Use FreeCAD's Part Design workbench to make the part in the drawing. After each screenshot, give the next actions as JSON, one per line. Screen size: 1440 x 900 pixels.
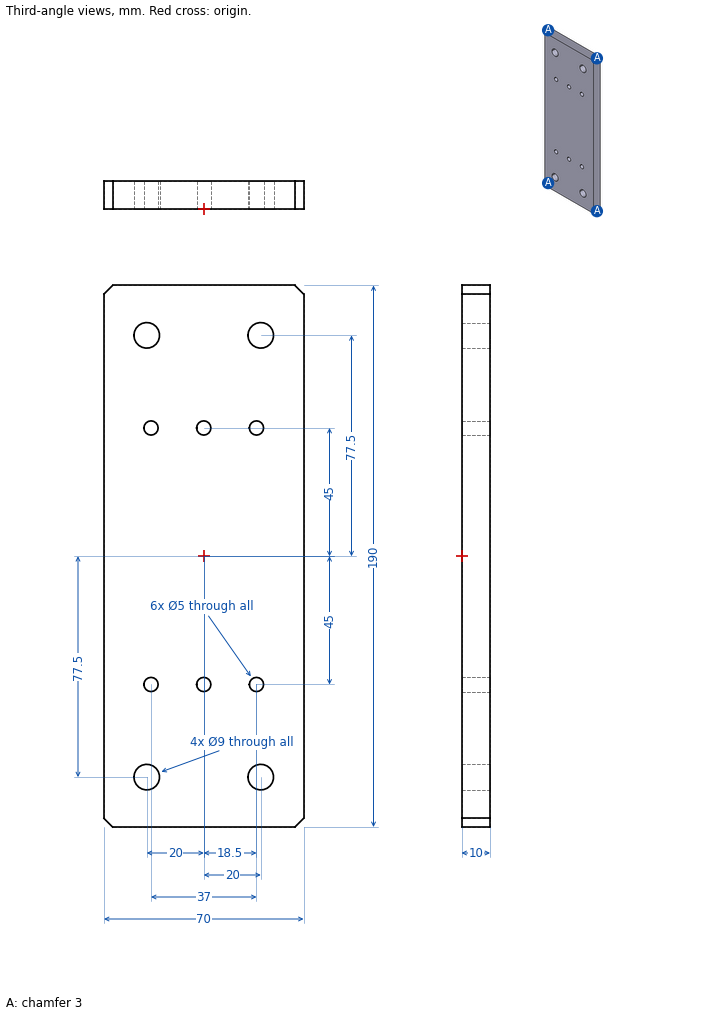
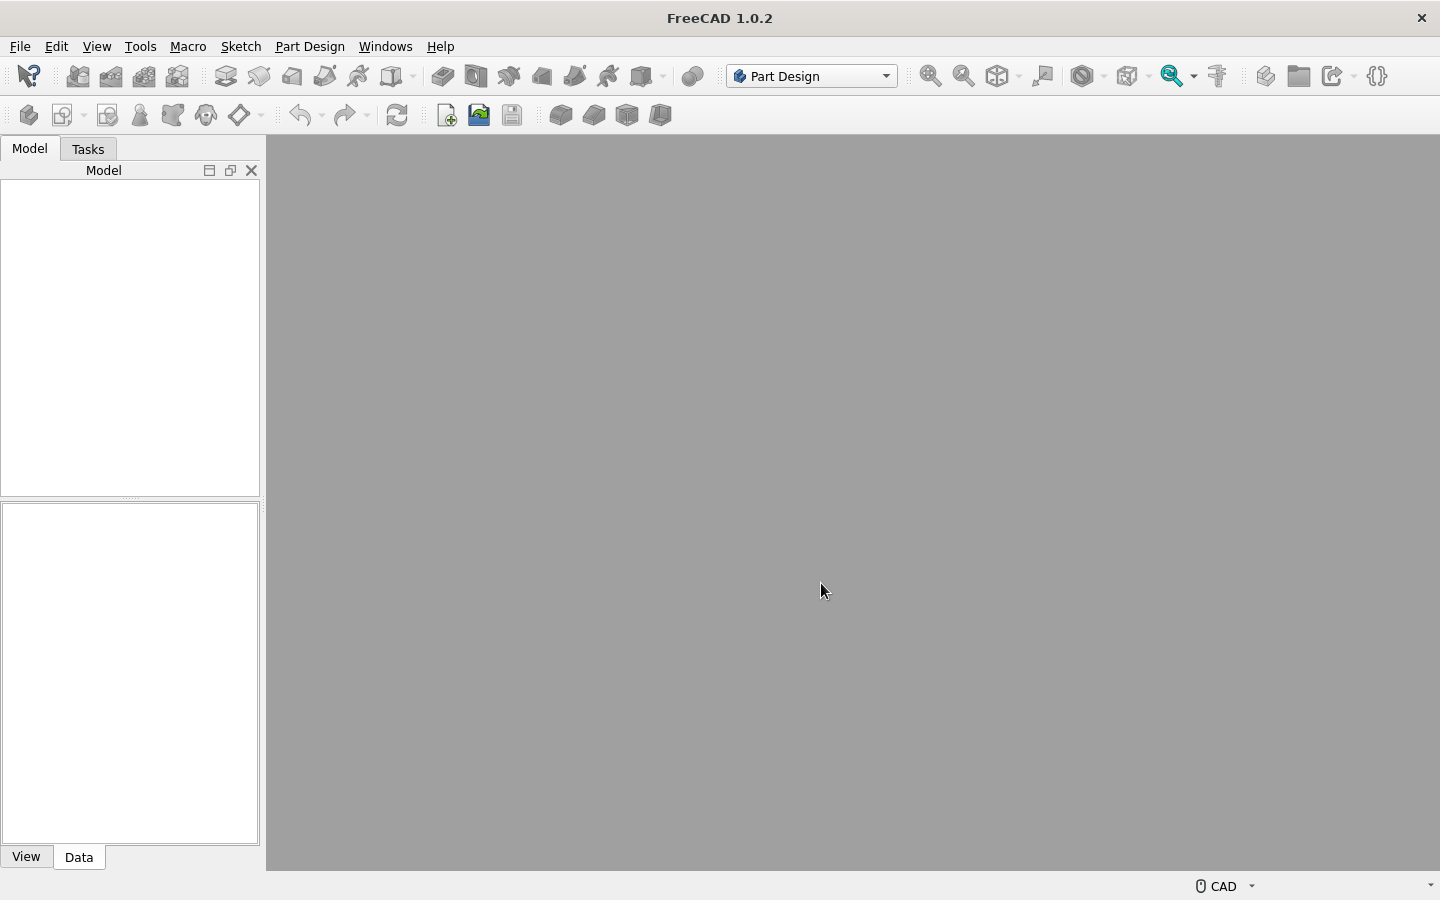
{"action": "left_click", "coordinate": [446, 116]}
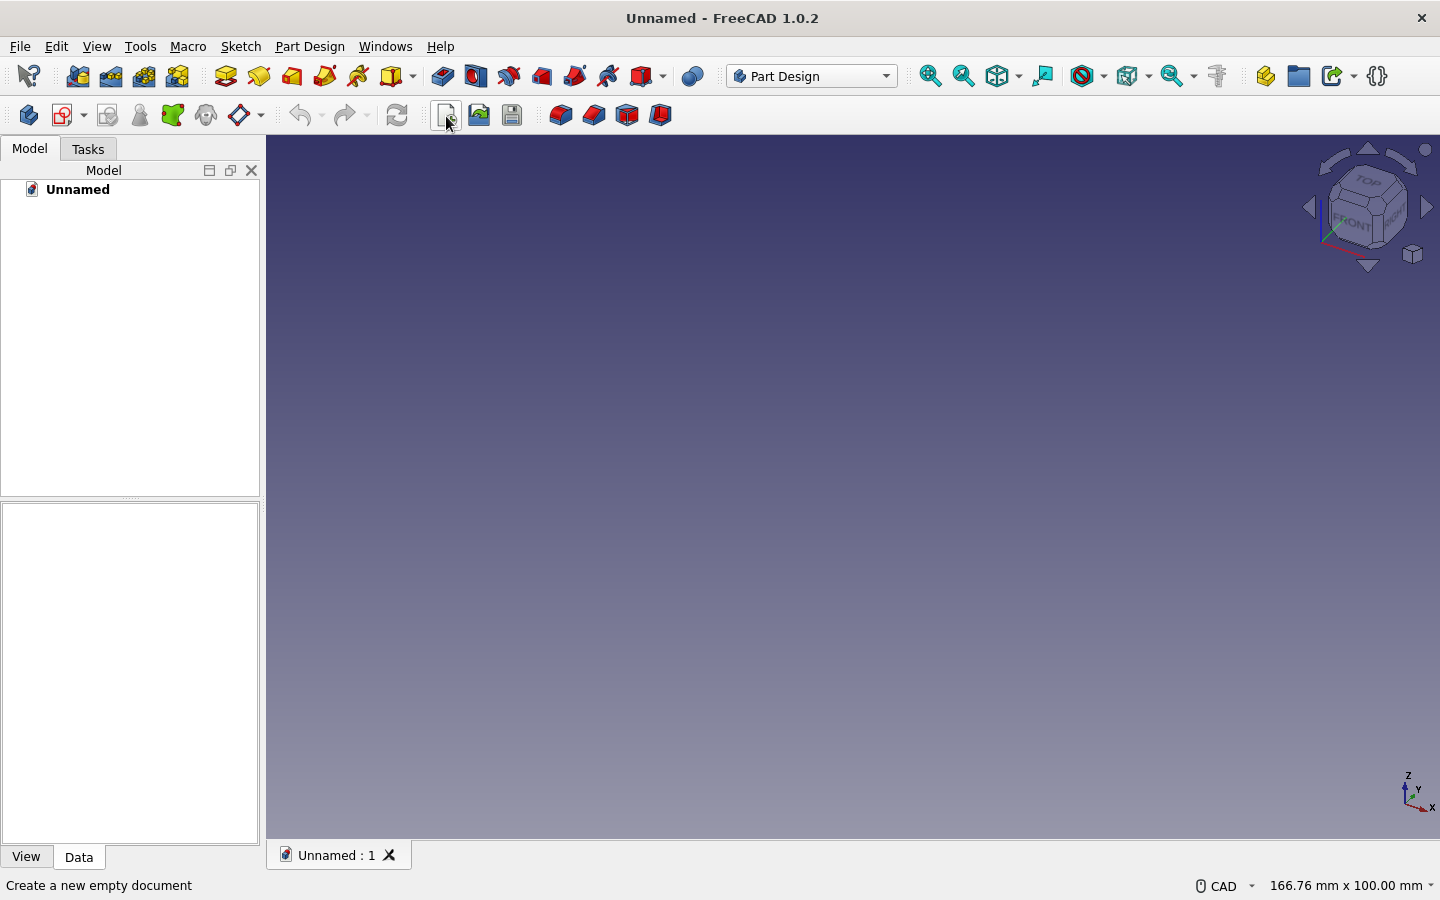
{"action": "left_click", "coordinate": [62, 116]}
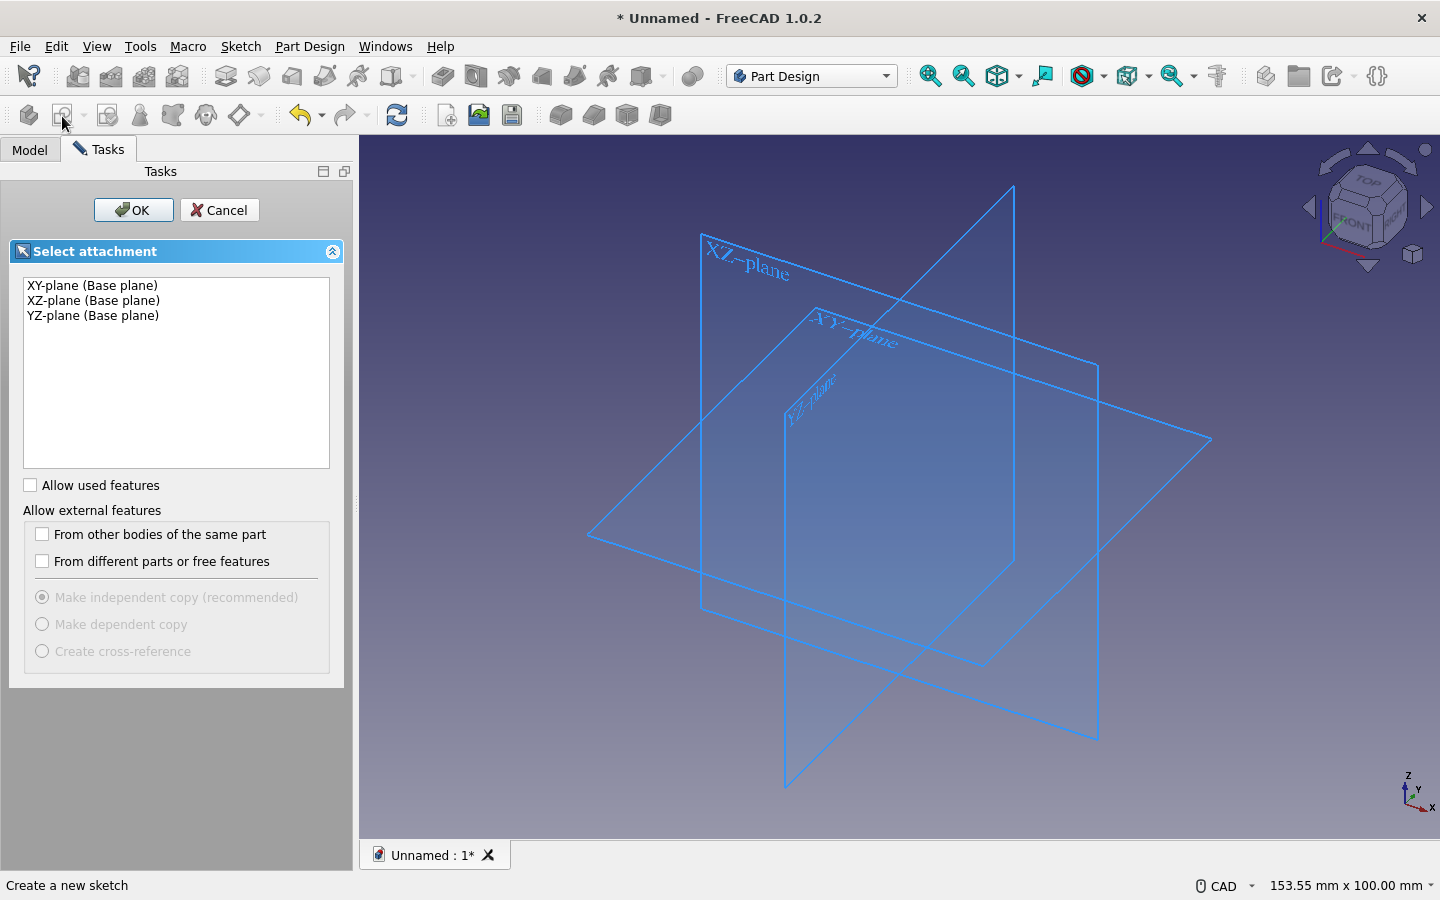
{"action": "left_click", "coordinate": [84, 300]}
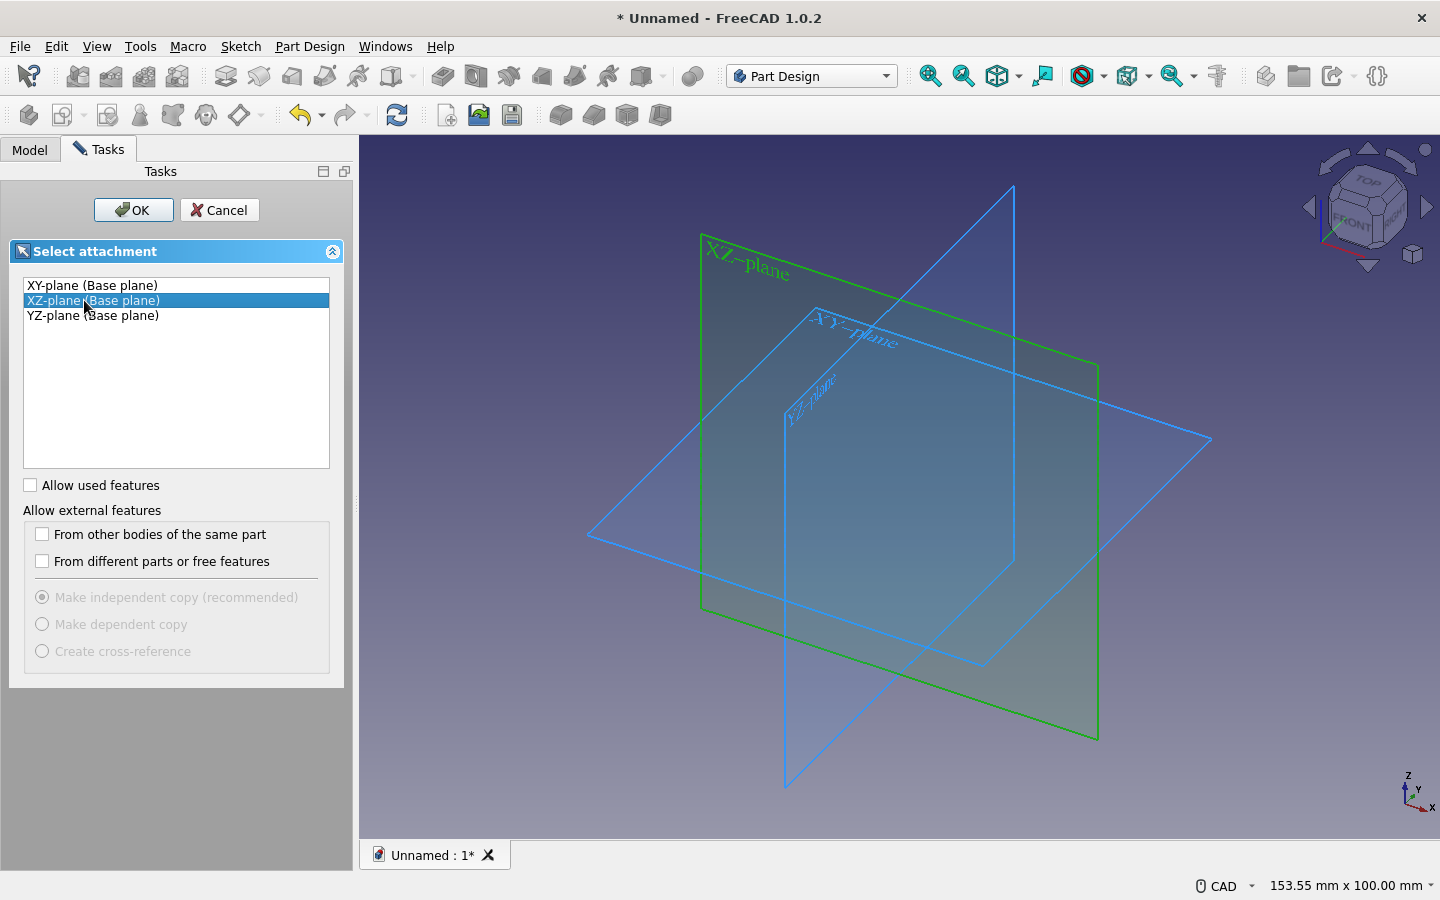
{"action": "left_click", "coordinate": [134, 210]}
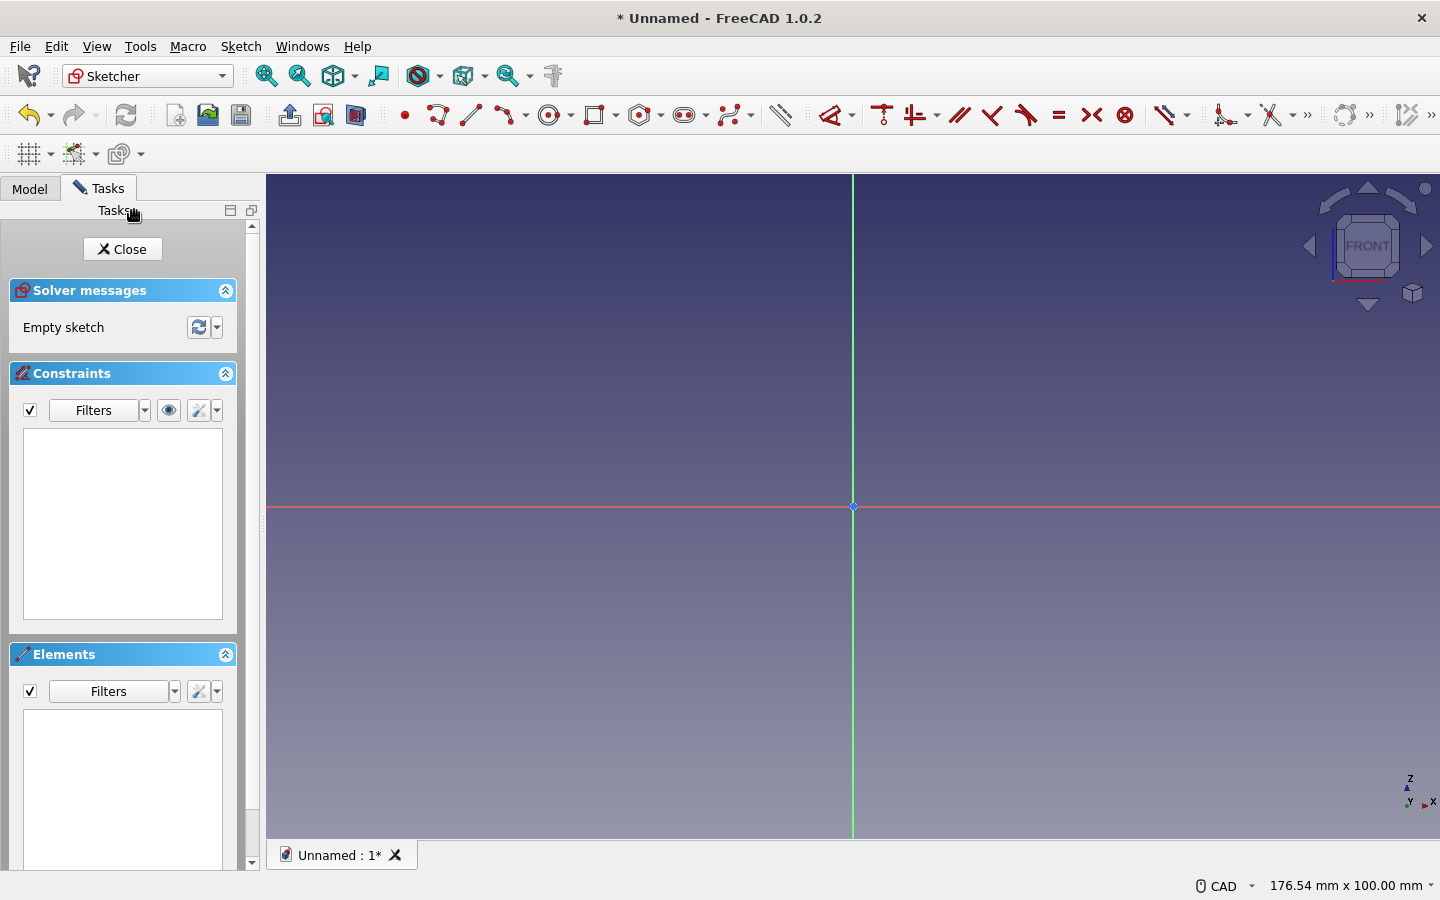
{"action": "scroll", "coordinate": [745, 506], "scroll_direction": "down", "scroll_amount": 5}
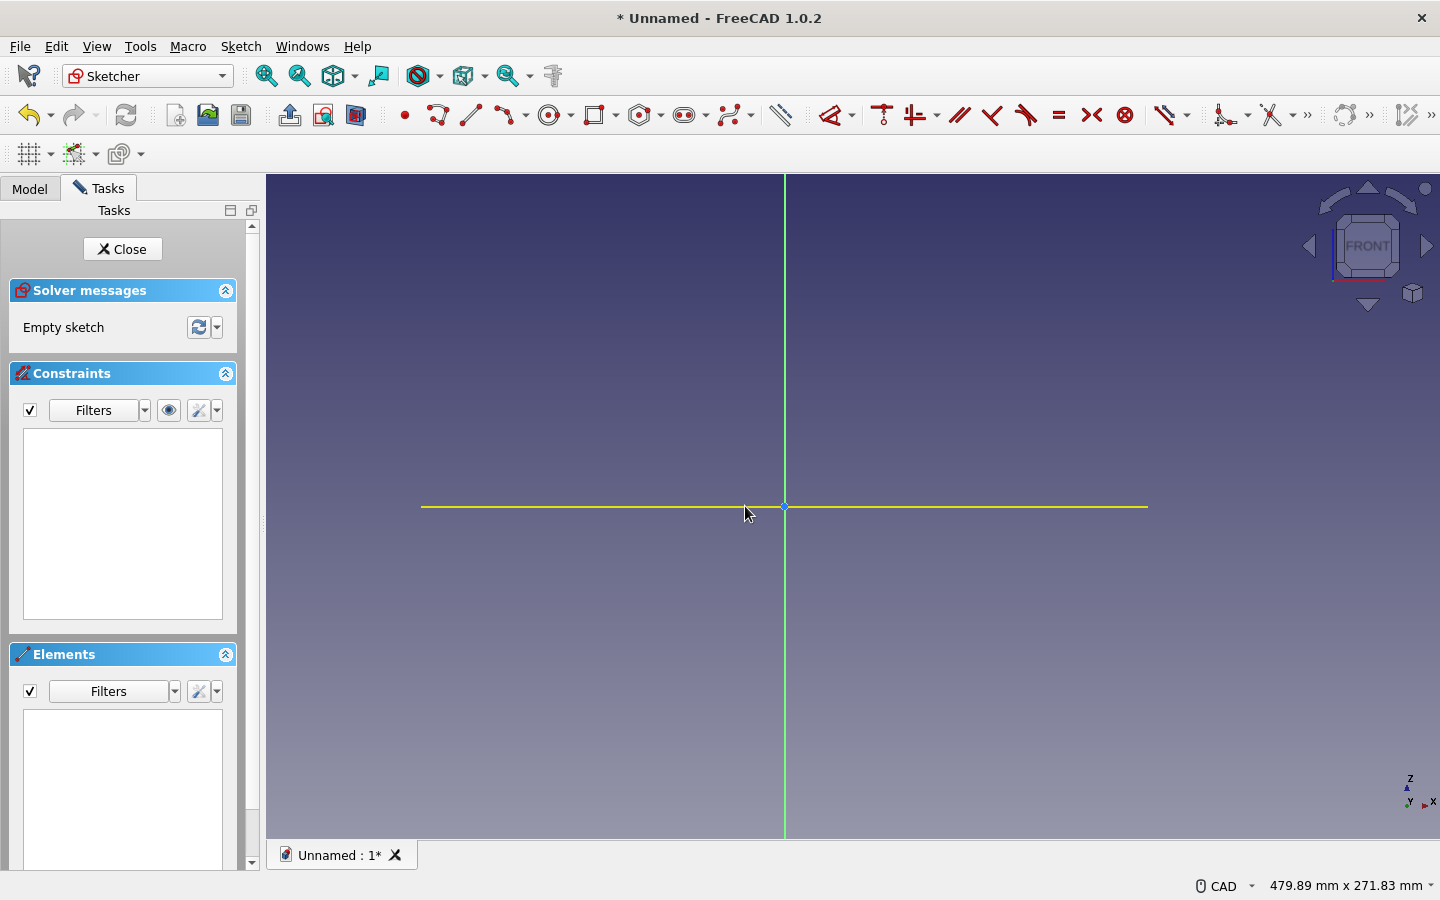
{"action": "left_click", "coordinate": [616, 116]}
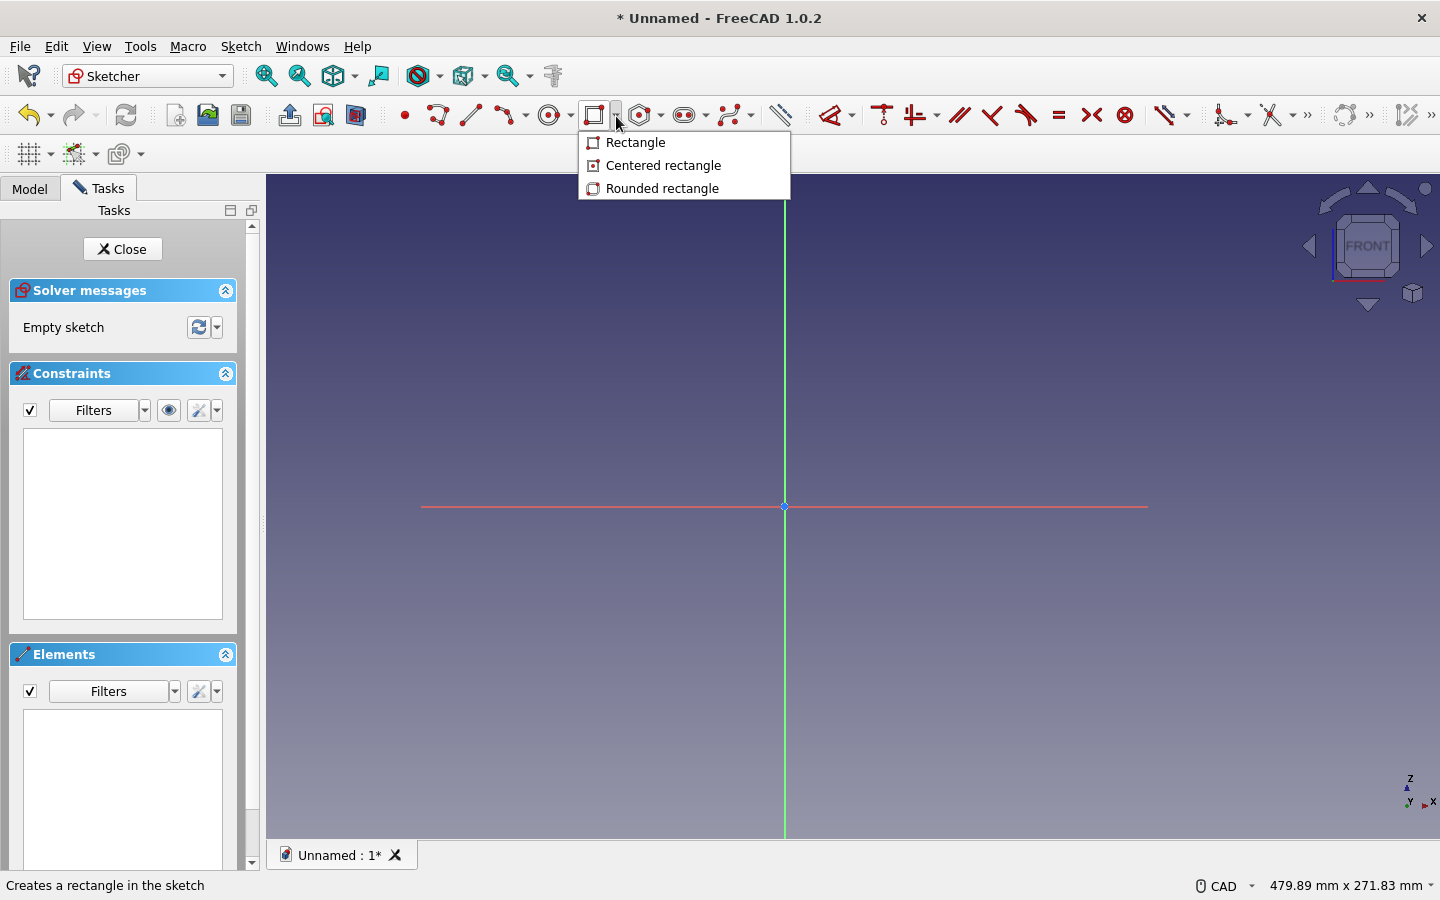
{"action": "left_click", "coordinate": [684, 166]}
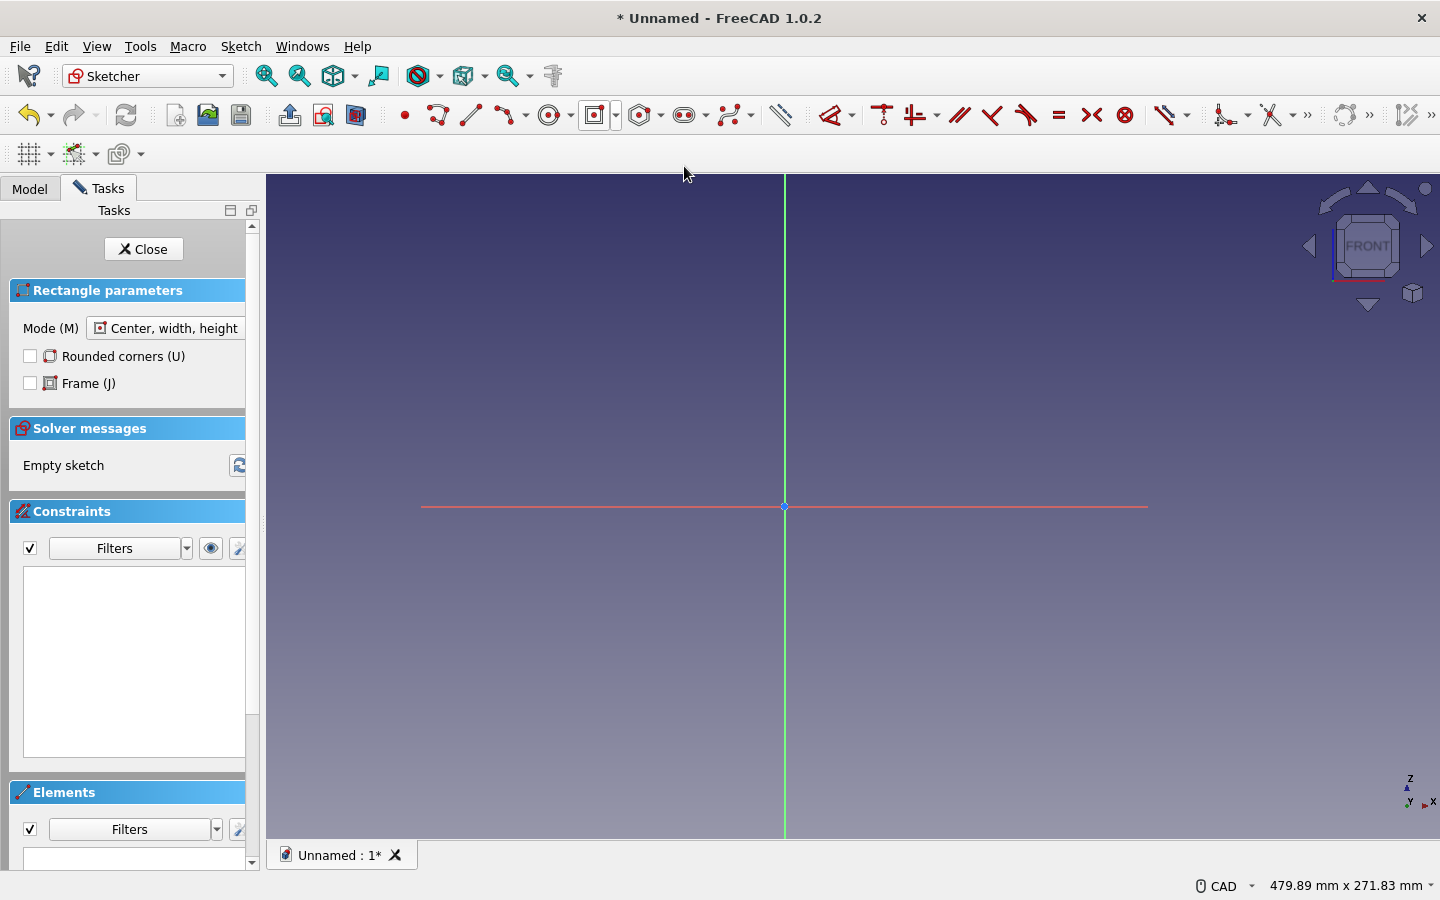
{"action": "left_click", "coordinate": [785, 506]}
{"action": "left_click", "coordinate": [871, 274]}
{"action": "key", "text": "Escape"}